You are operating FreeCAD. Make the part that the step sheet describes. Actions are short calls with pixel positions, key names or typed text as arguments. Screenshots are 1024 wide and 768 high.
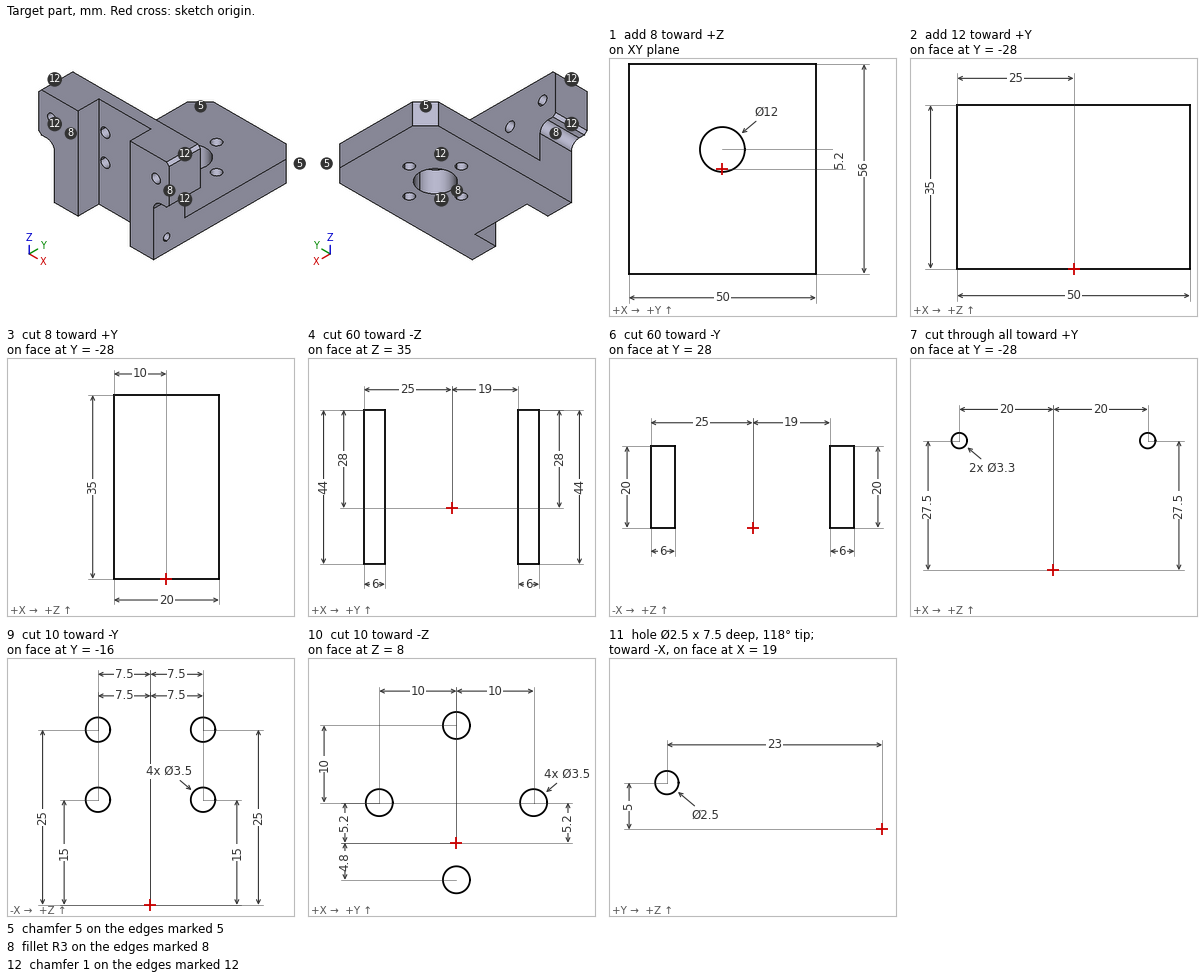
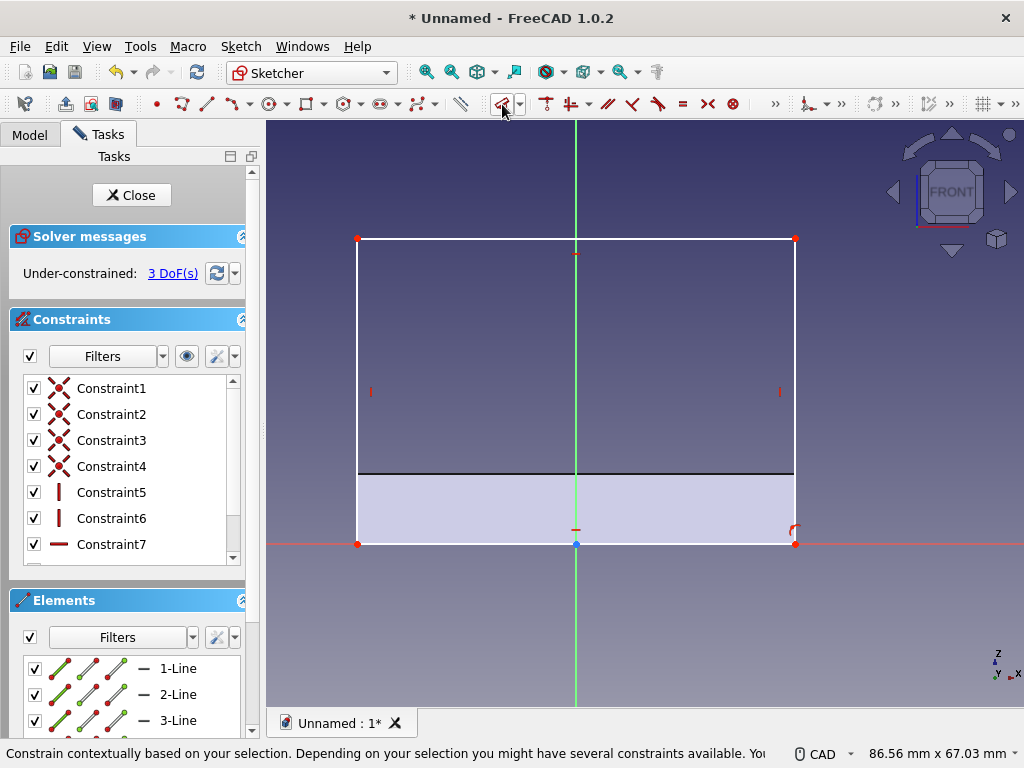
click(357, 331)
click(323, 392)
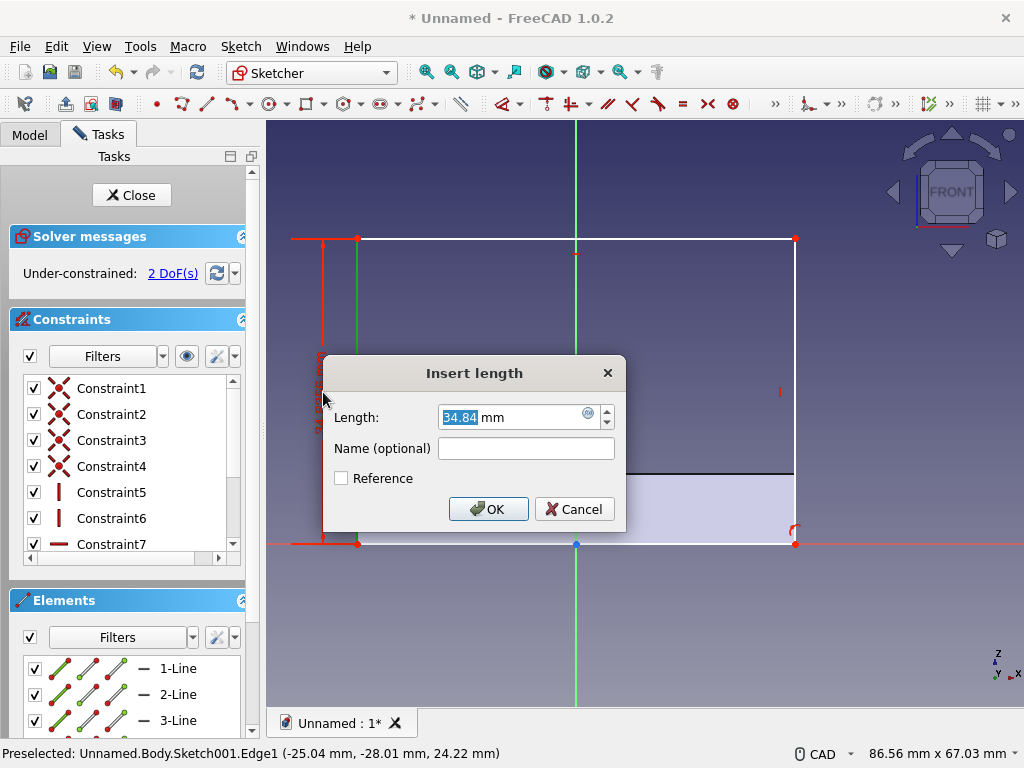
text(35)
key(Return)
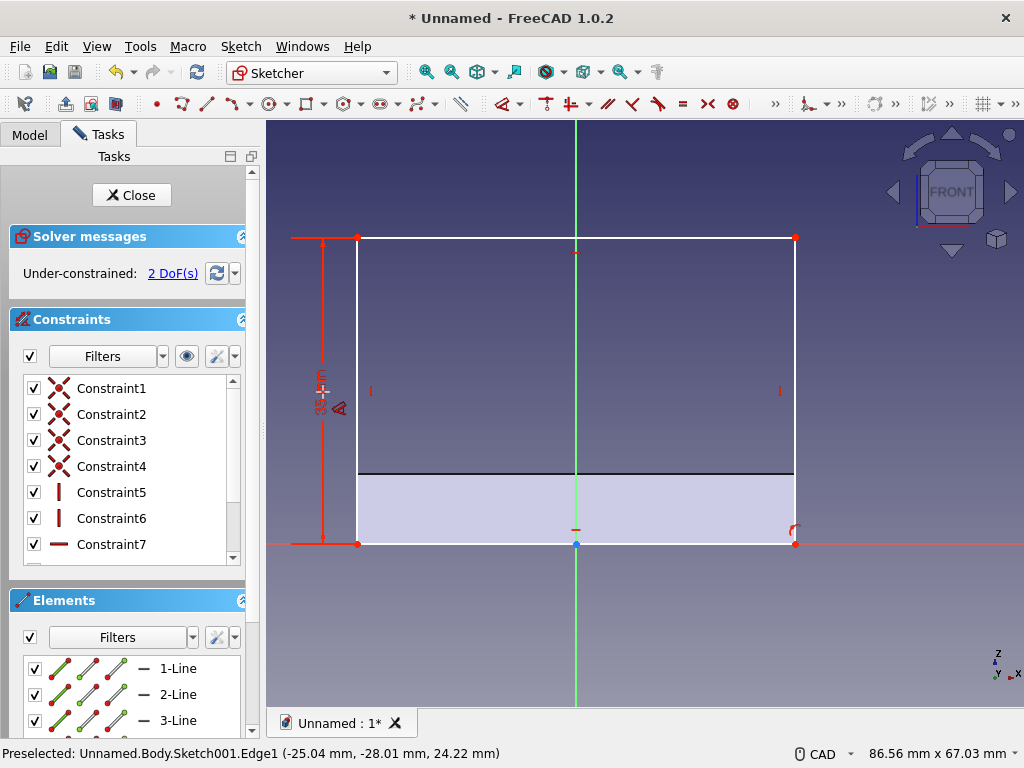
click(488, 544)
click(475, 578)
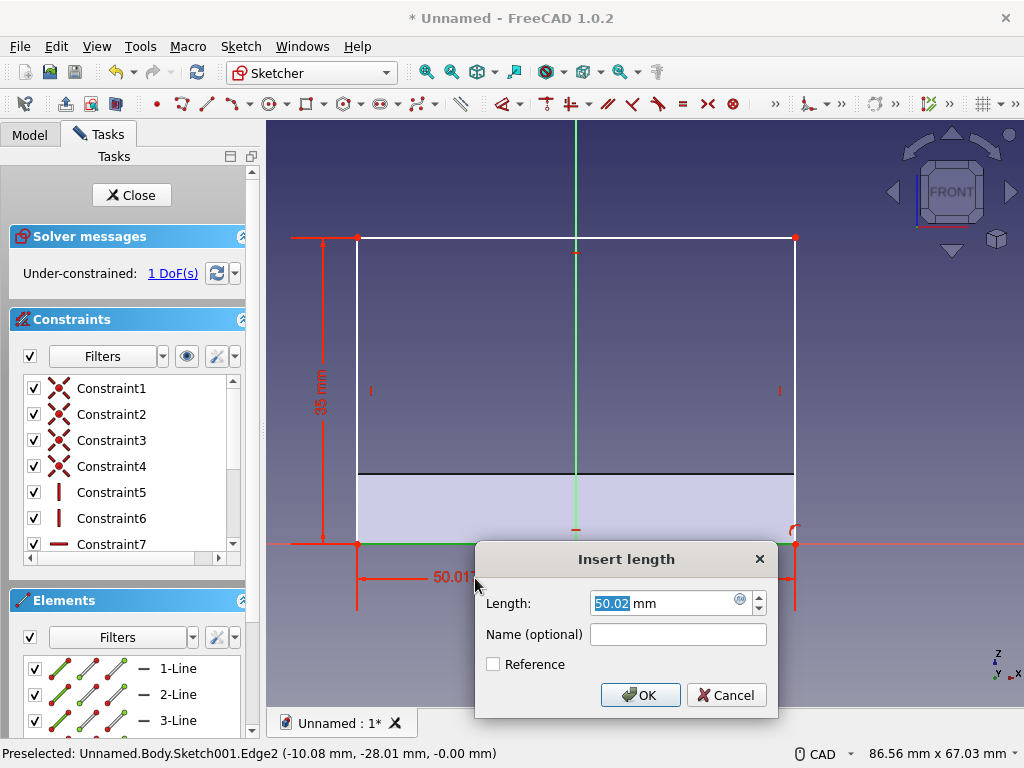
text(50)
key(Return)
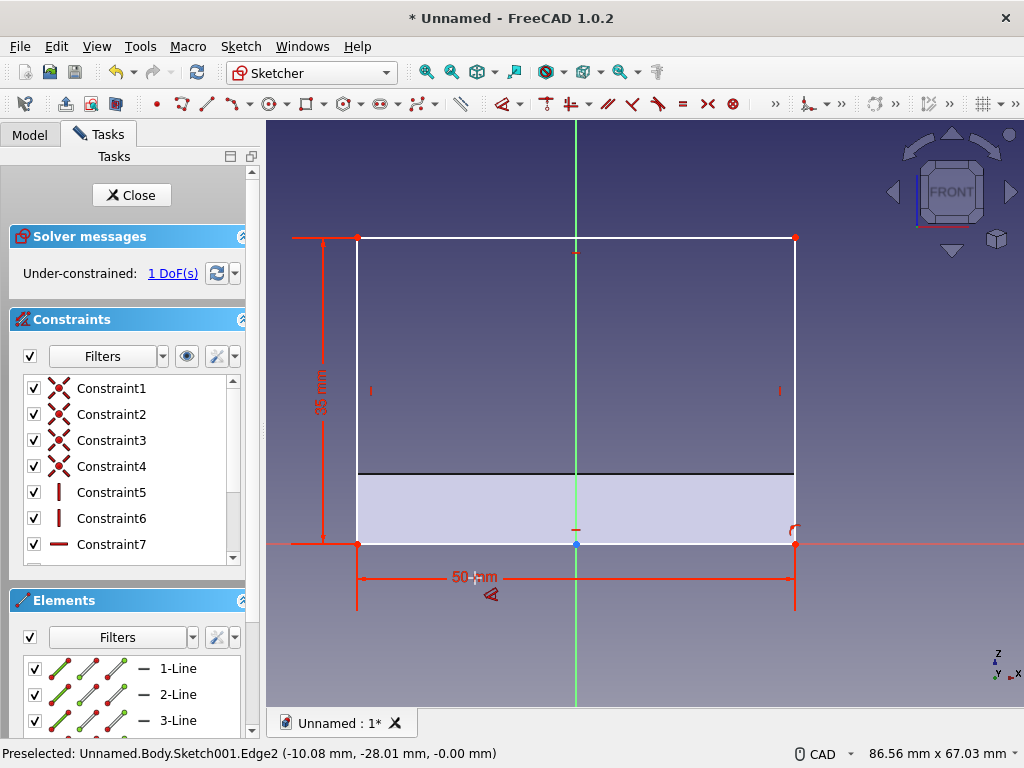
click(357, 238)
click(390, 578)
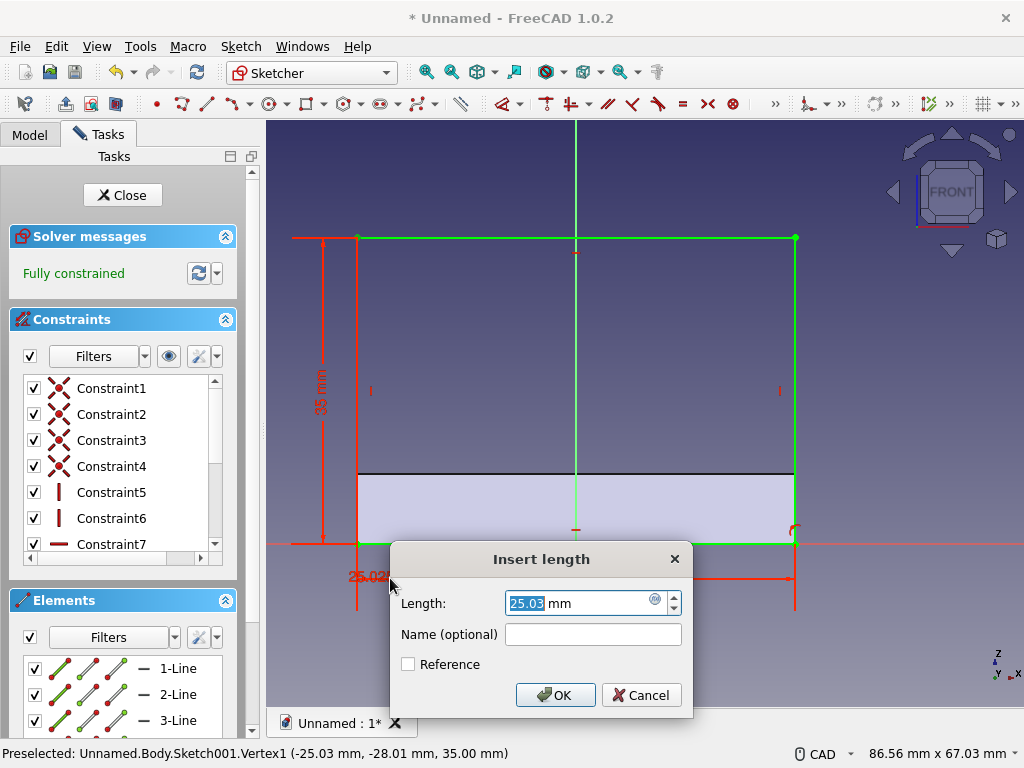
text(25)
key(Return)
key(Escape)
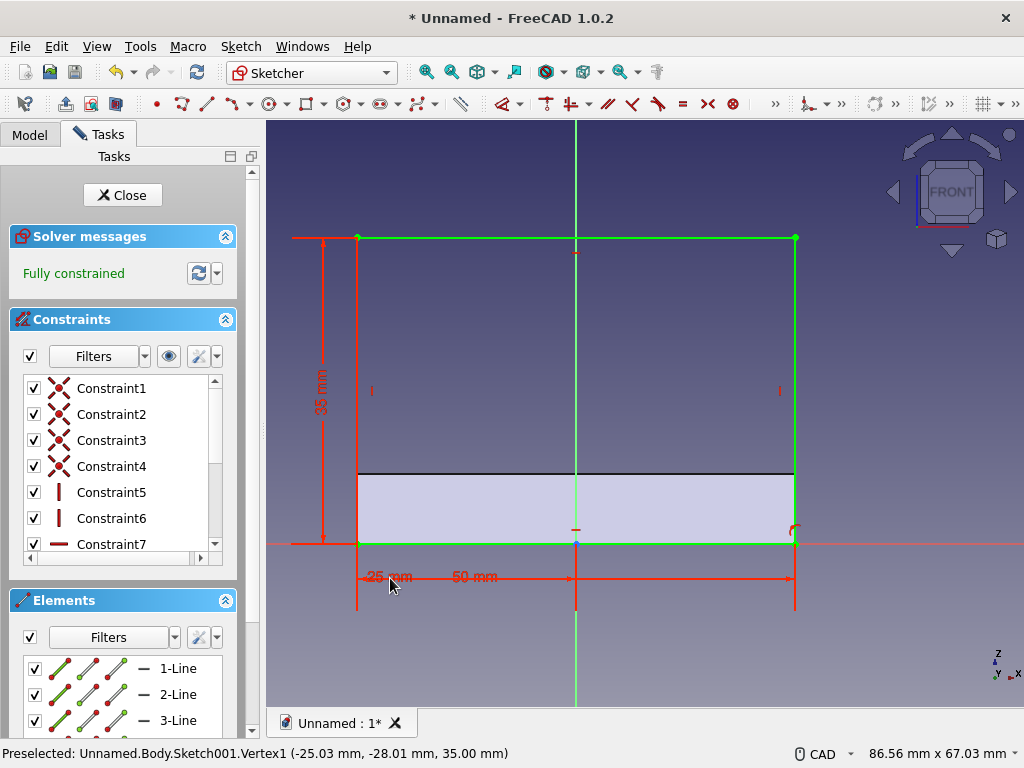
click(123, 195)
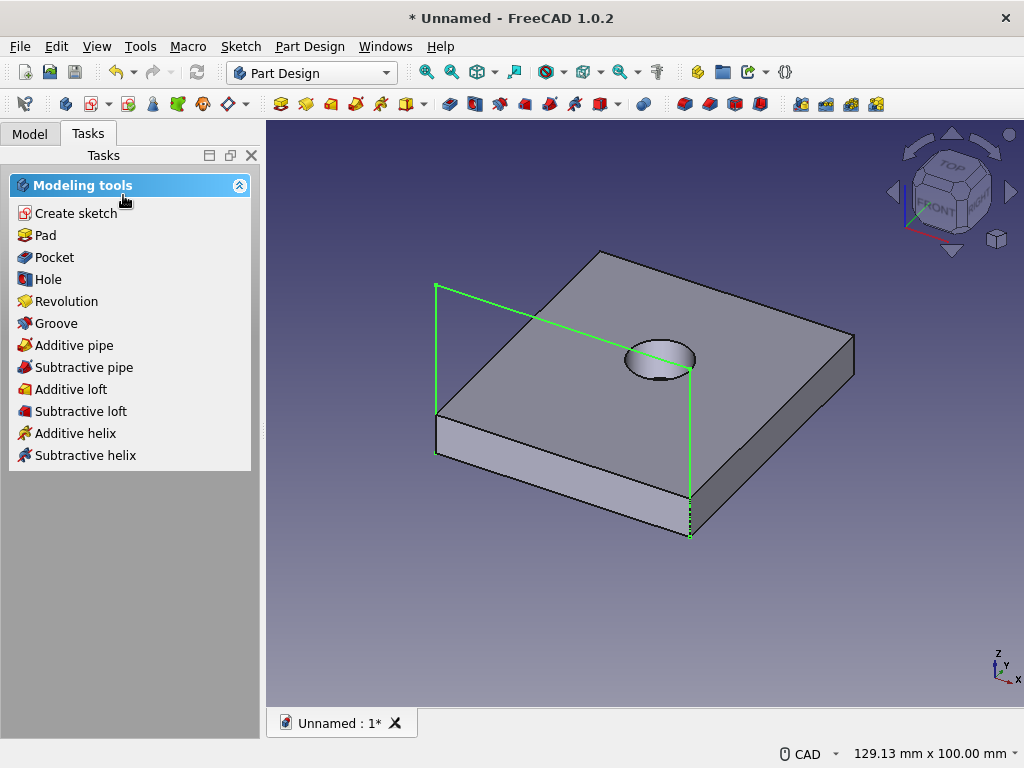
click(281, 104)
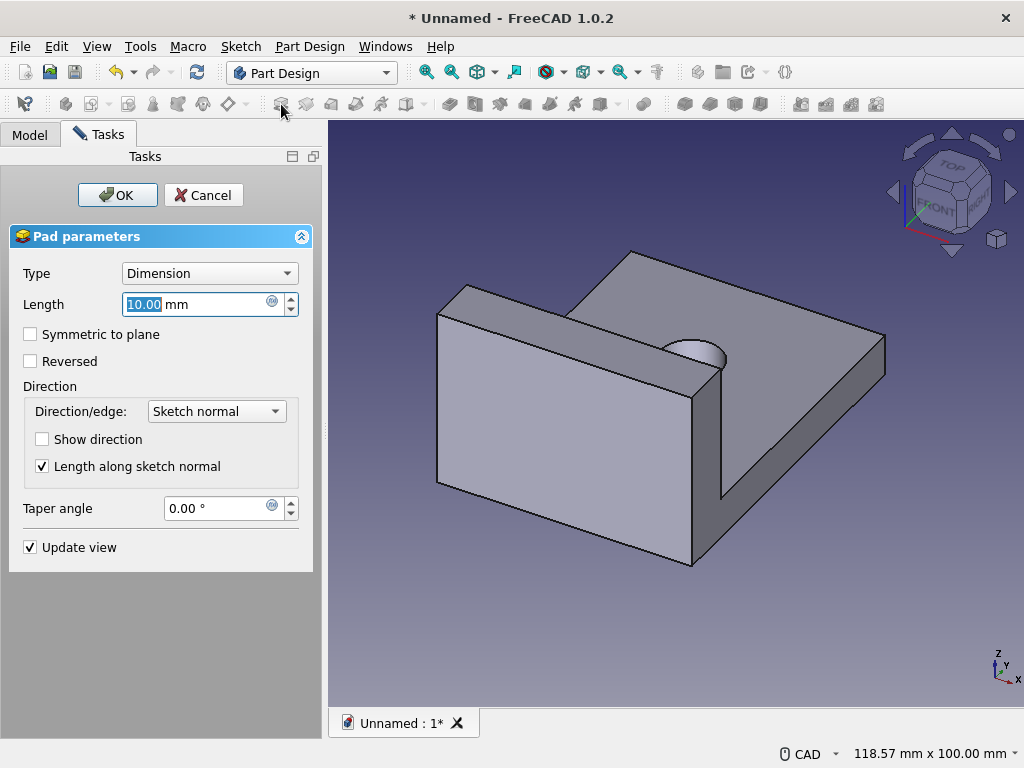
text(12)
key(Tab)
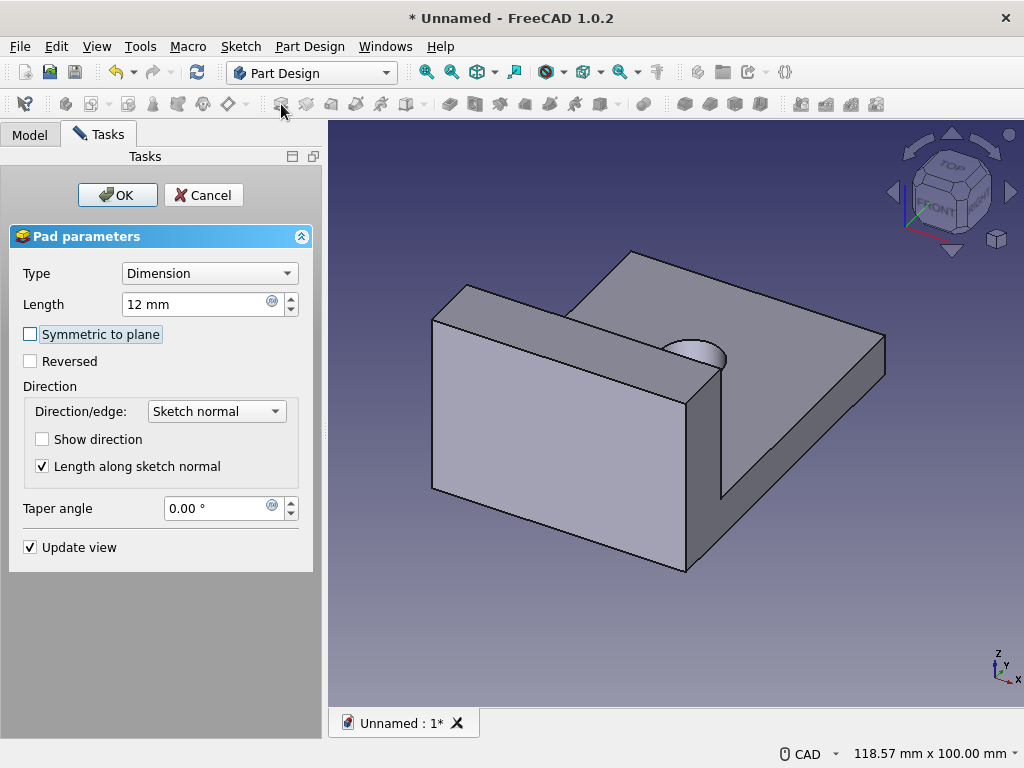
click(31, 361)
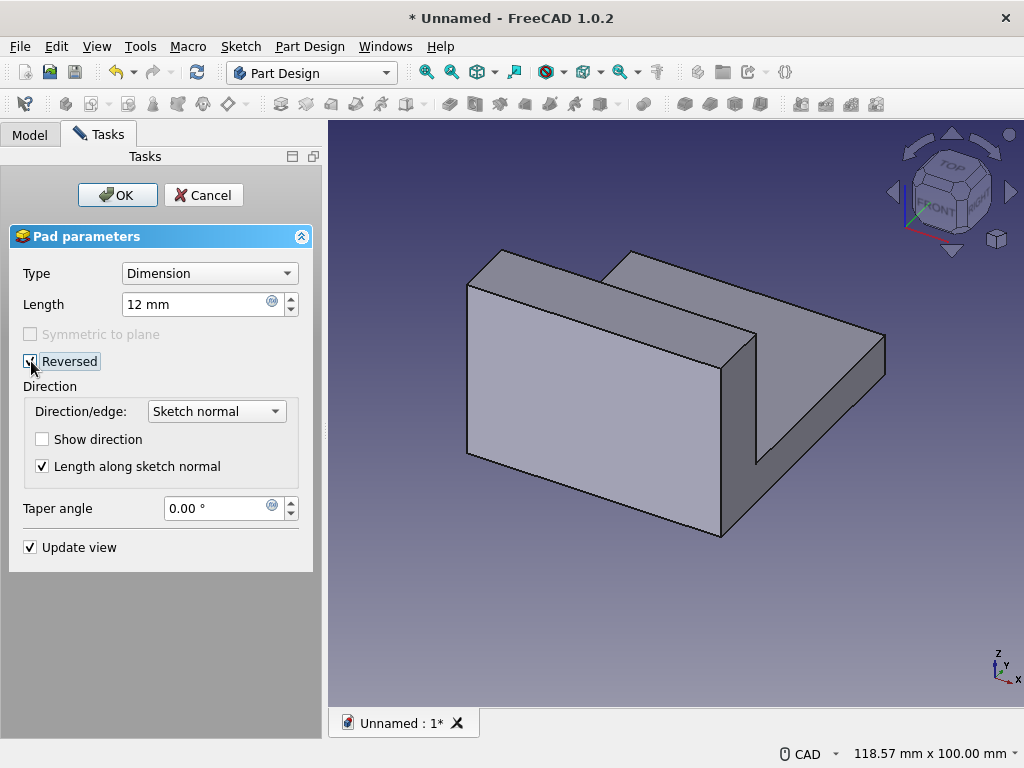
click(118, 195)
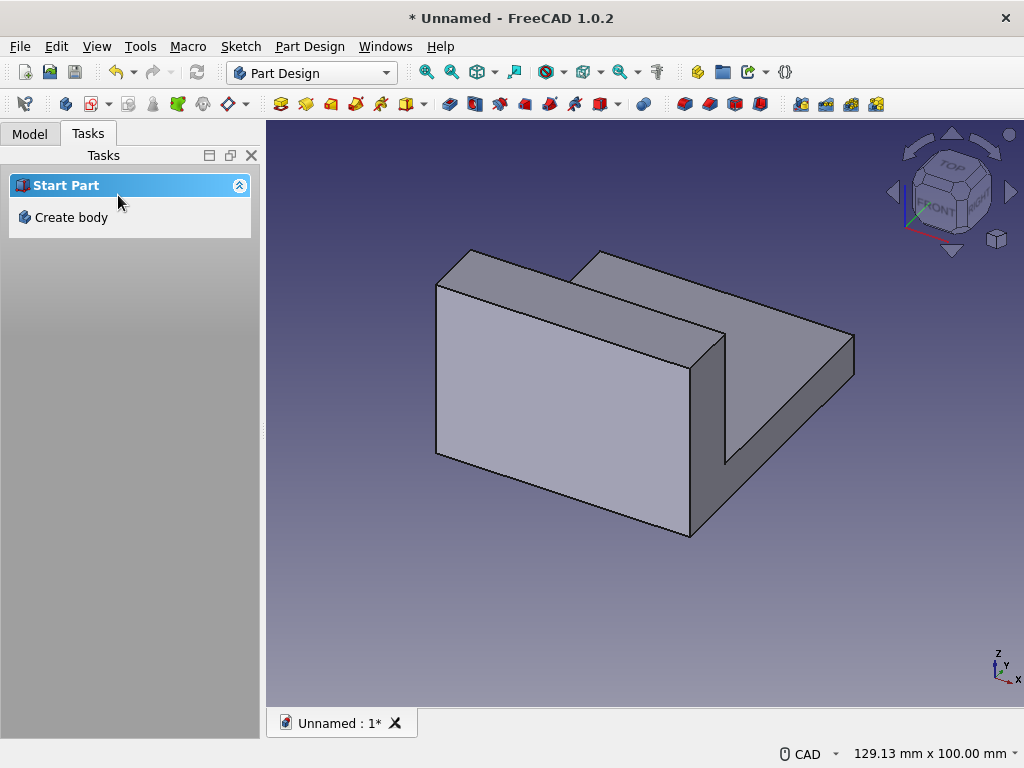
click(599, 422)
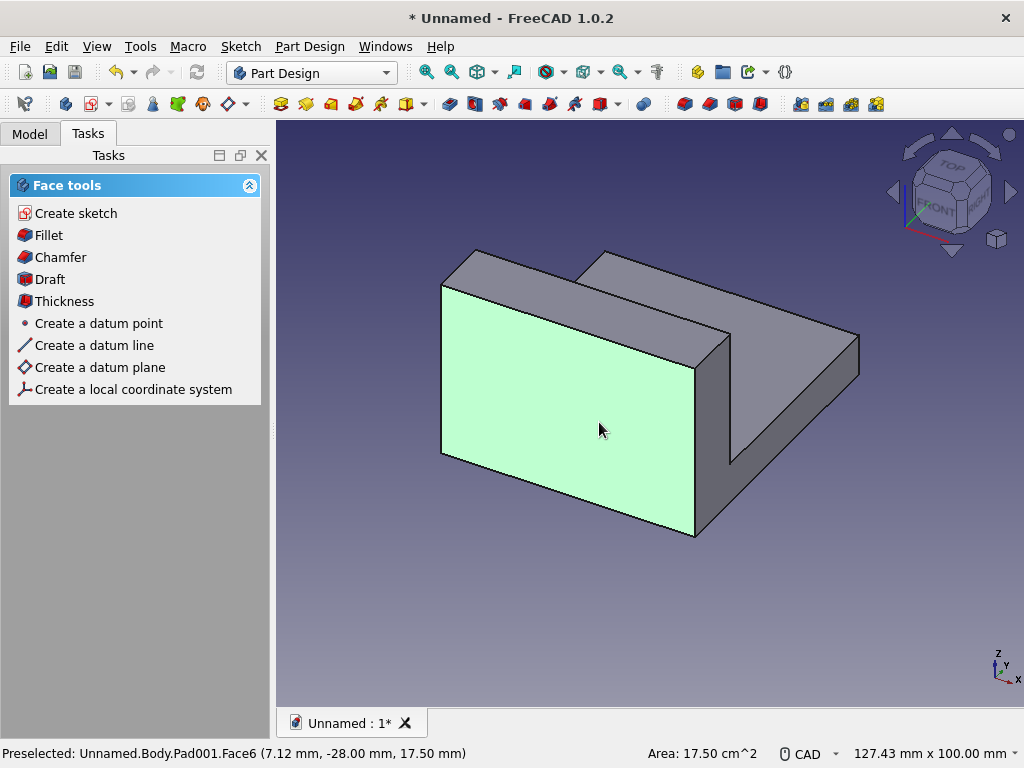
click(90, 104)